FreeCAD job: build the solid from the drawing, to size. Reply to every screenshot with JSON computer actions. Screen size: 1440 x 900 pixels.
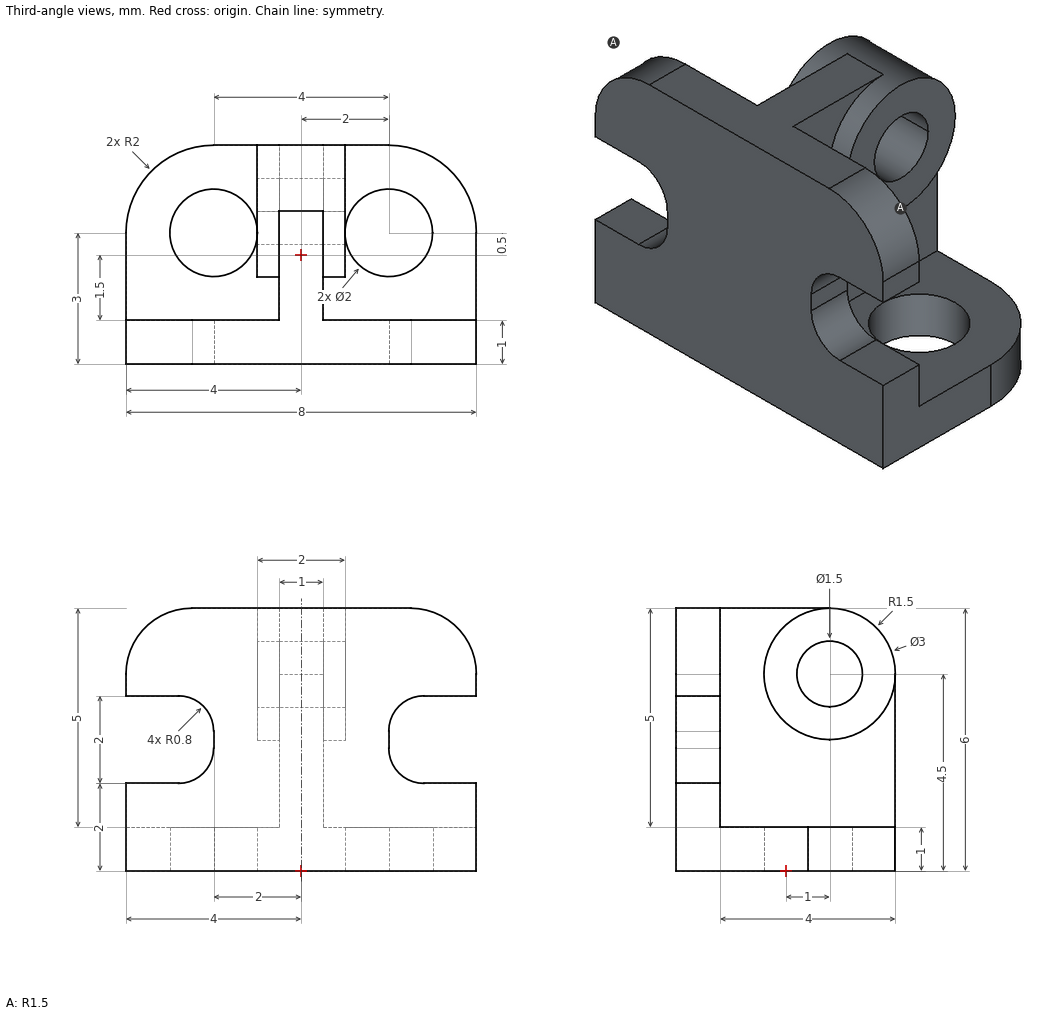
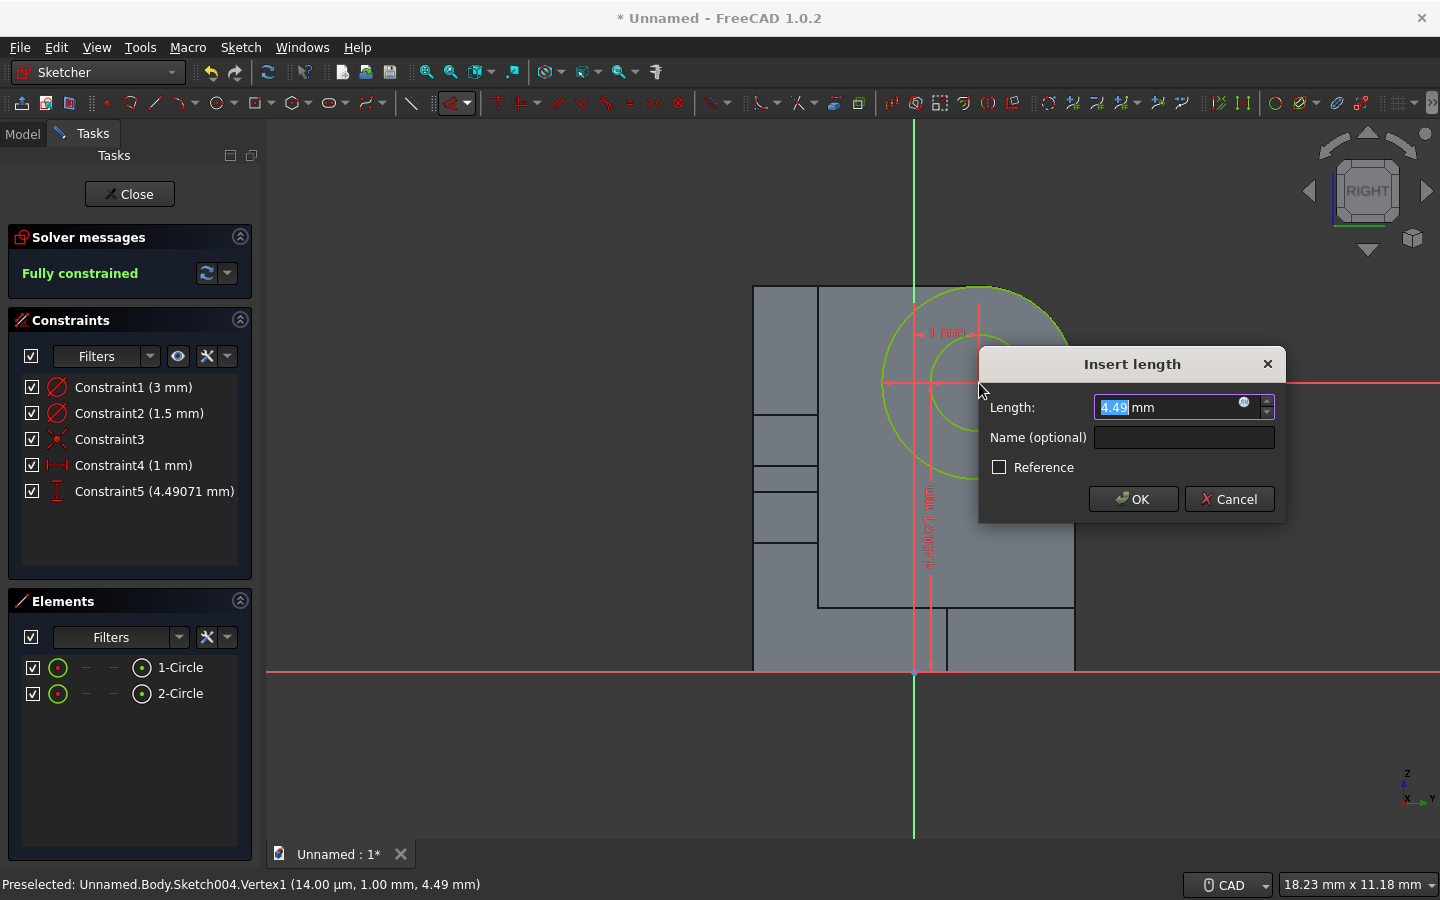
{"action": "type", "text": "4.5"}
{"action": "key", "text": "Return"}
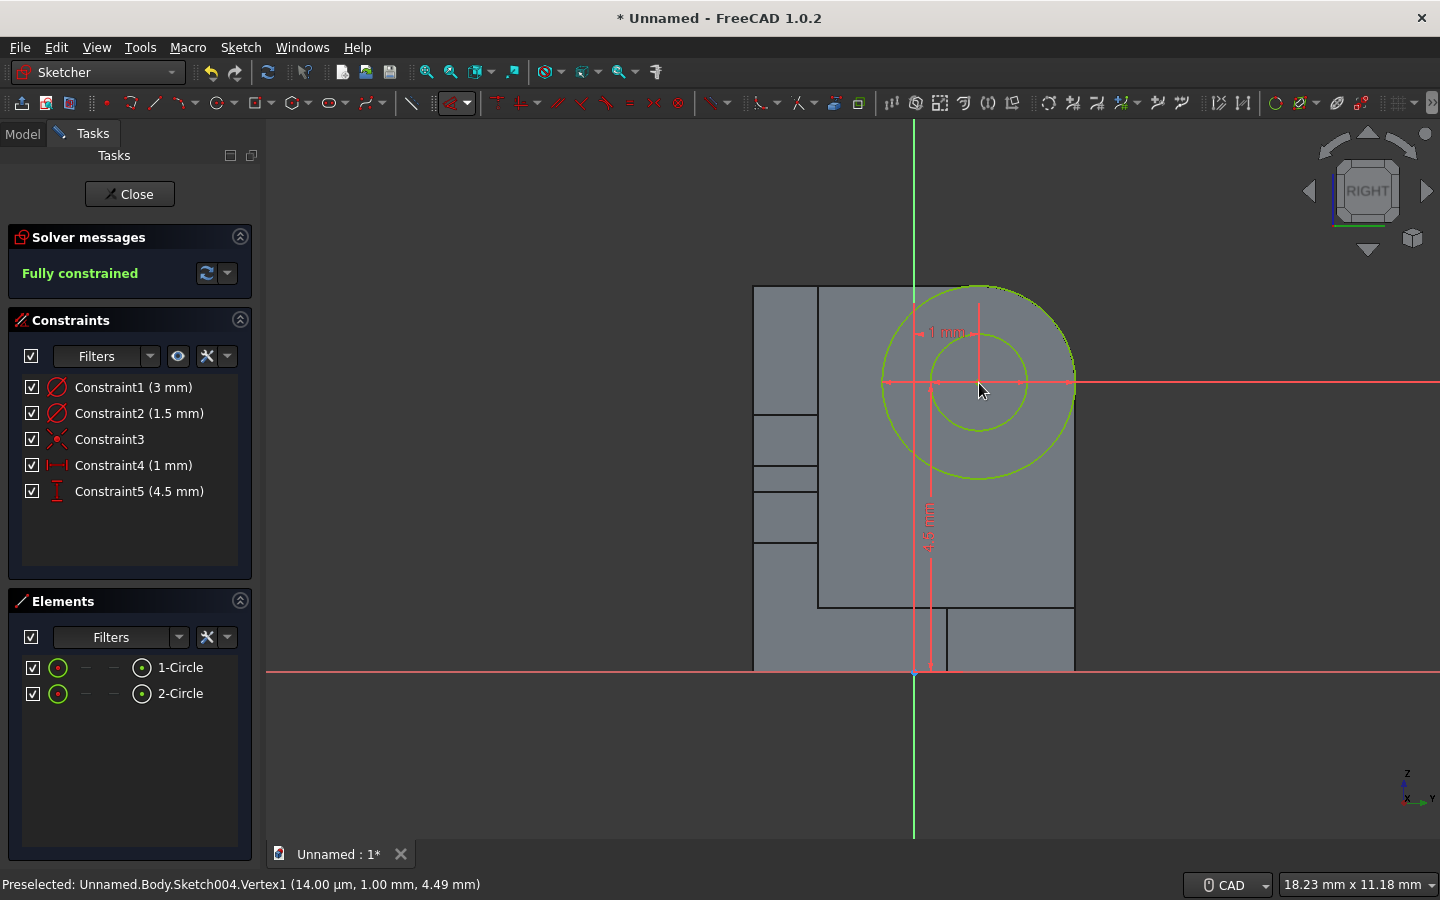
{"action": "left_click", "coordinate": [130, 194]}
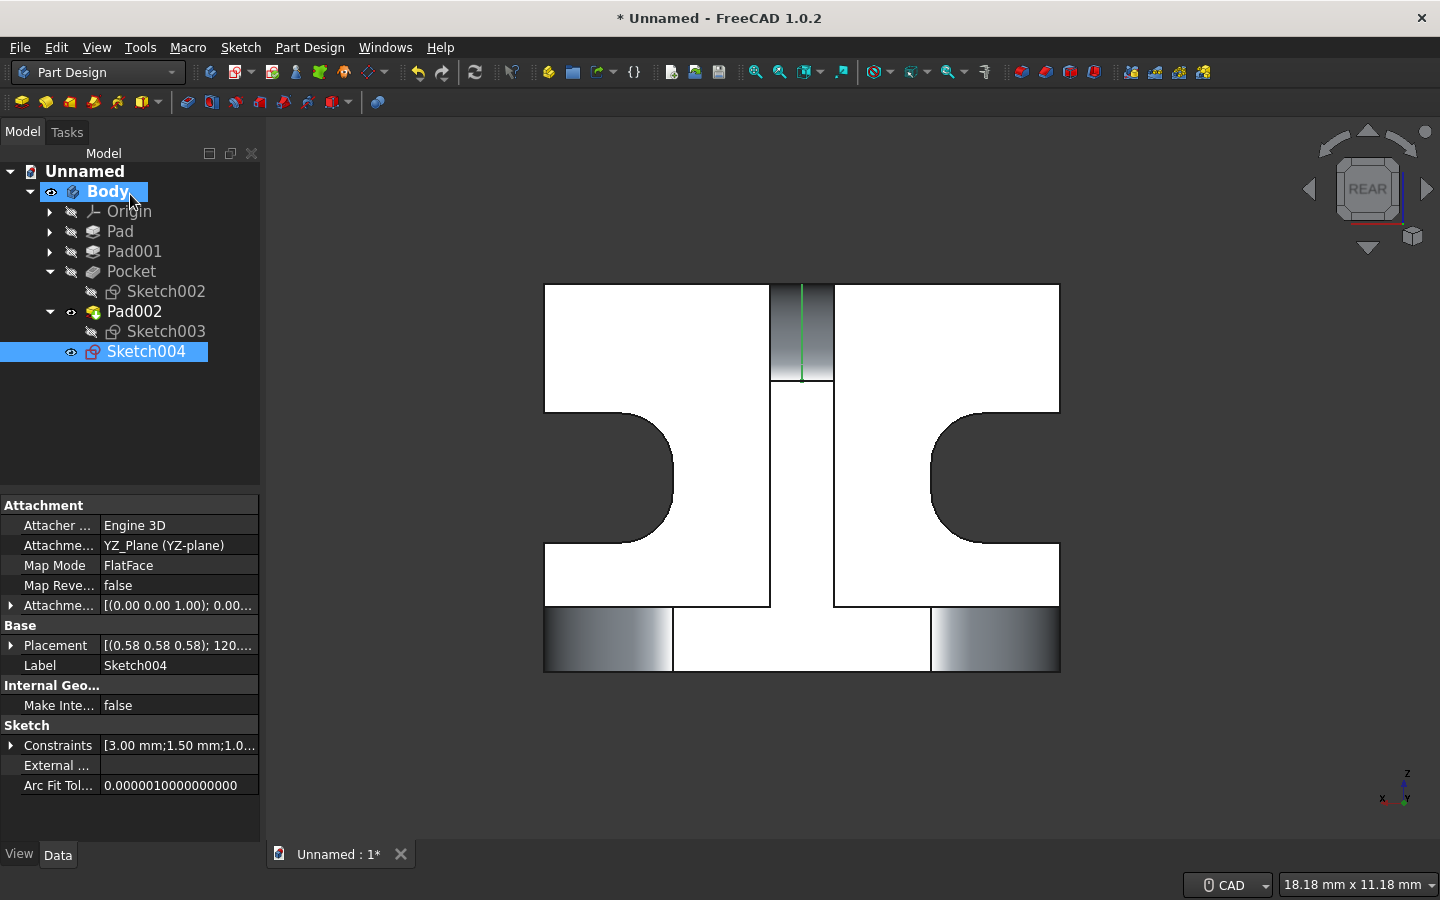
{"action": "left_click", "coordinate": [22, 102]}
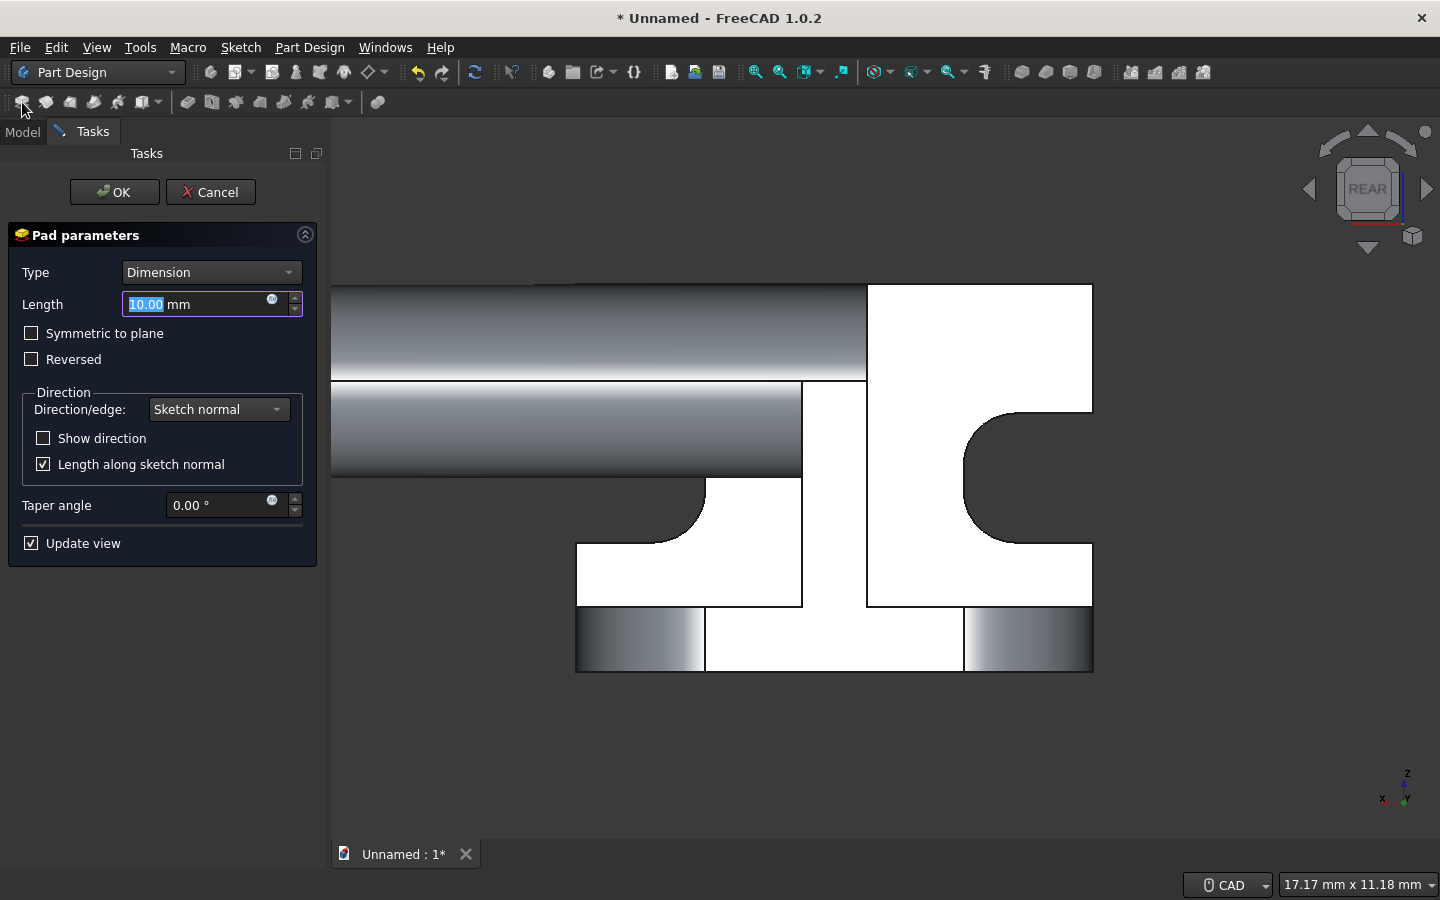
{"action": "type", "text": "2"}
{"action": "key", "text": "Tab"}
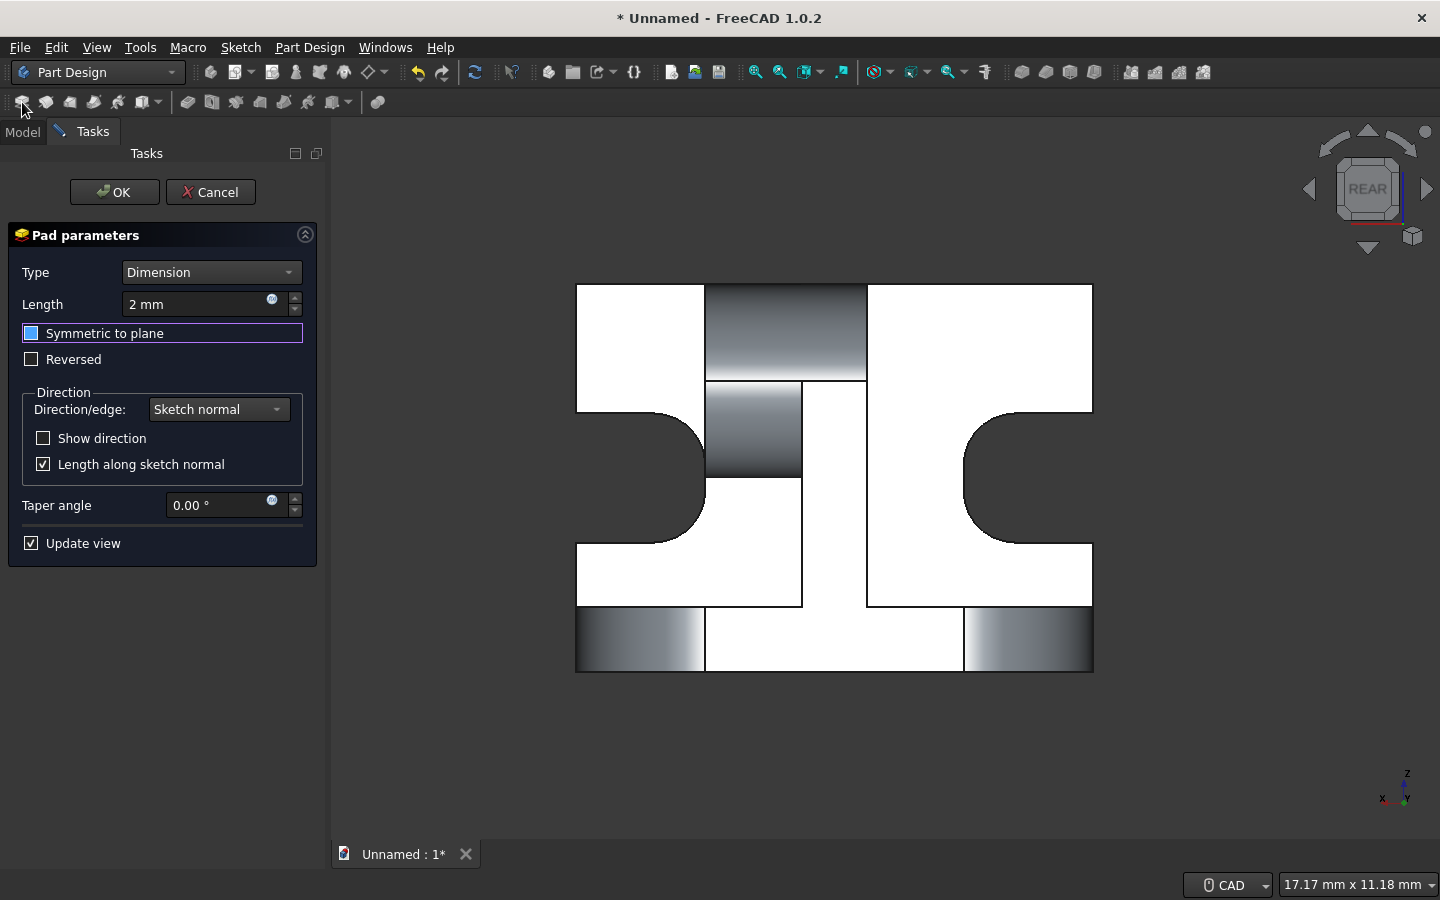
{"action": "left_click", "coordinate": [30, 333]}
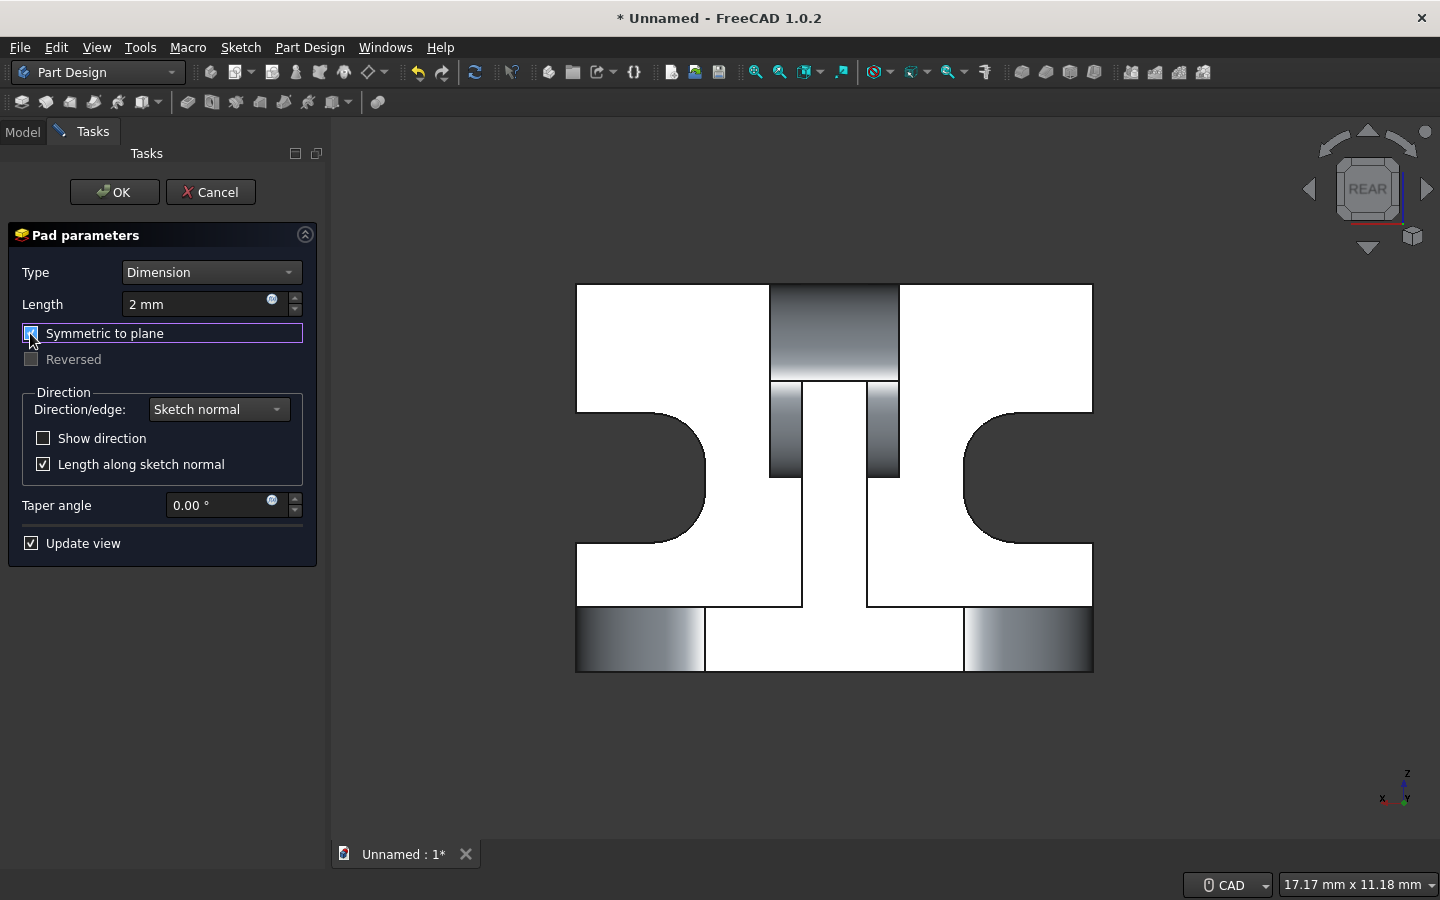
{"action": "left_click", "coordinate": [115, 192]}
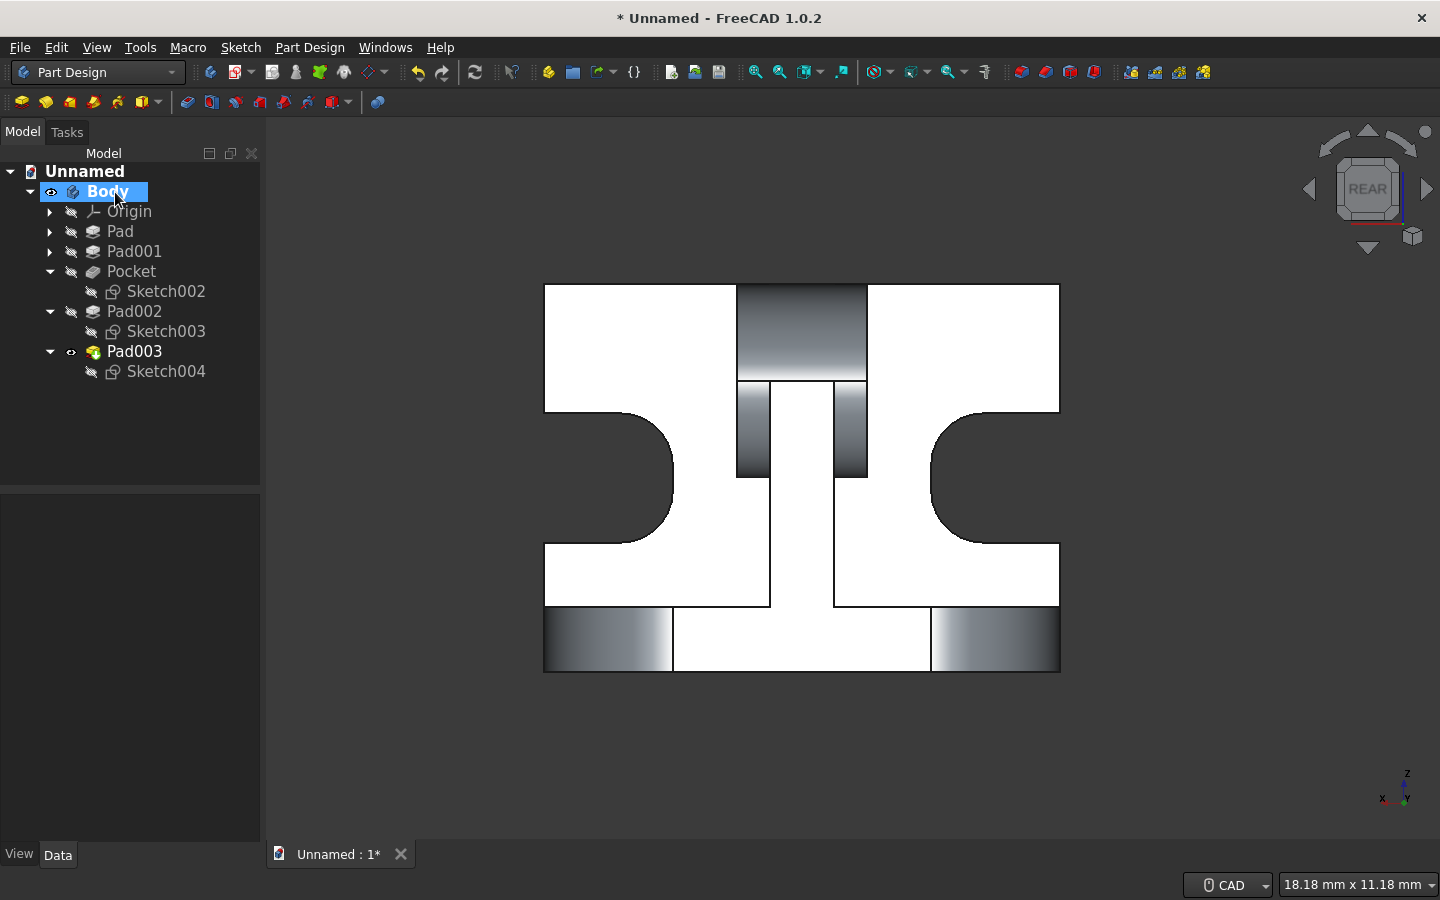
{"action": "key", "text": "0"}